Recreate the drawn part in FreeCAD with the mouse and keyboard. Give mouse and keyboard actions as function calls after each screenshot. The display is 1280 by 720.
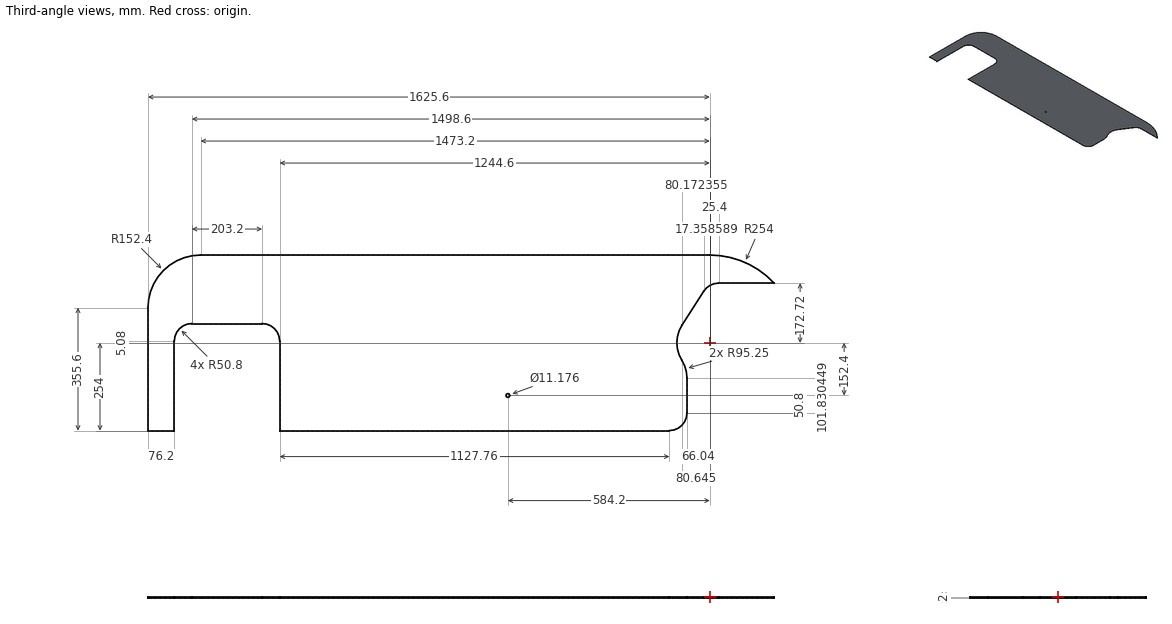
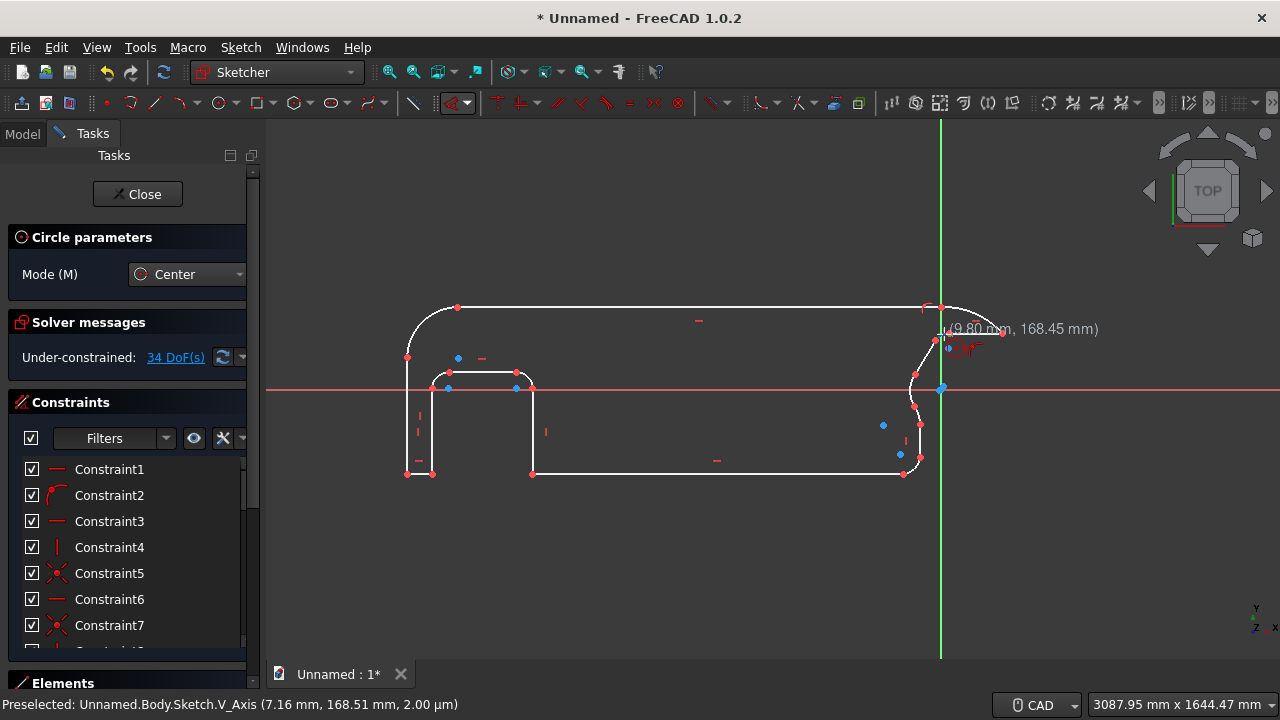
scroll(750, 440, up, 13)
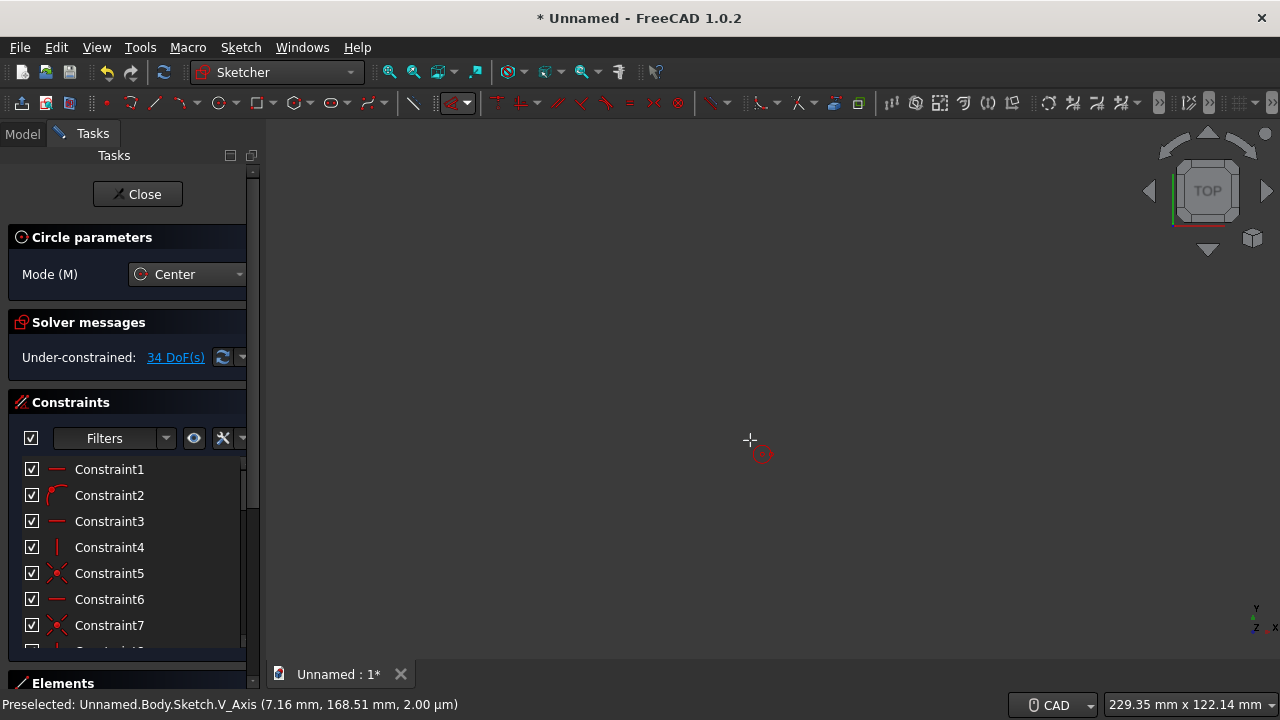
scroll(750, 440, down, 13)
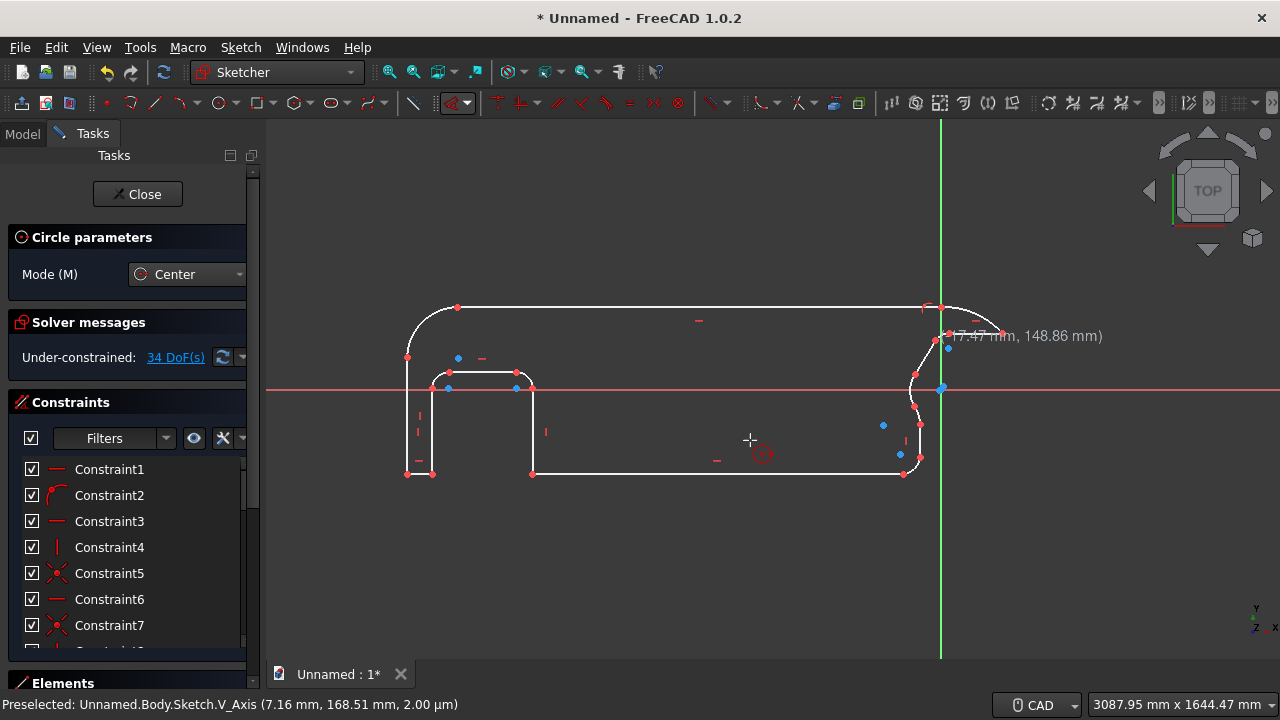
click(750, 440)
move(751, 439)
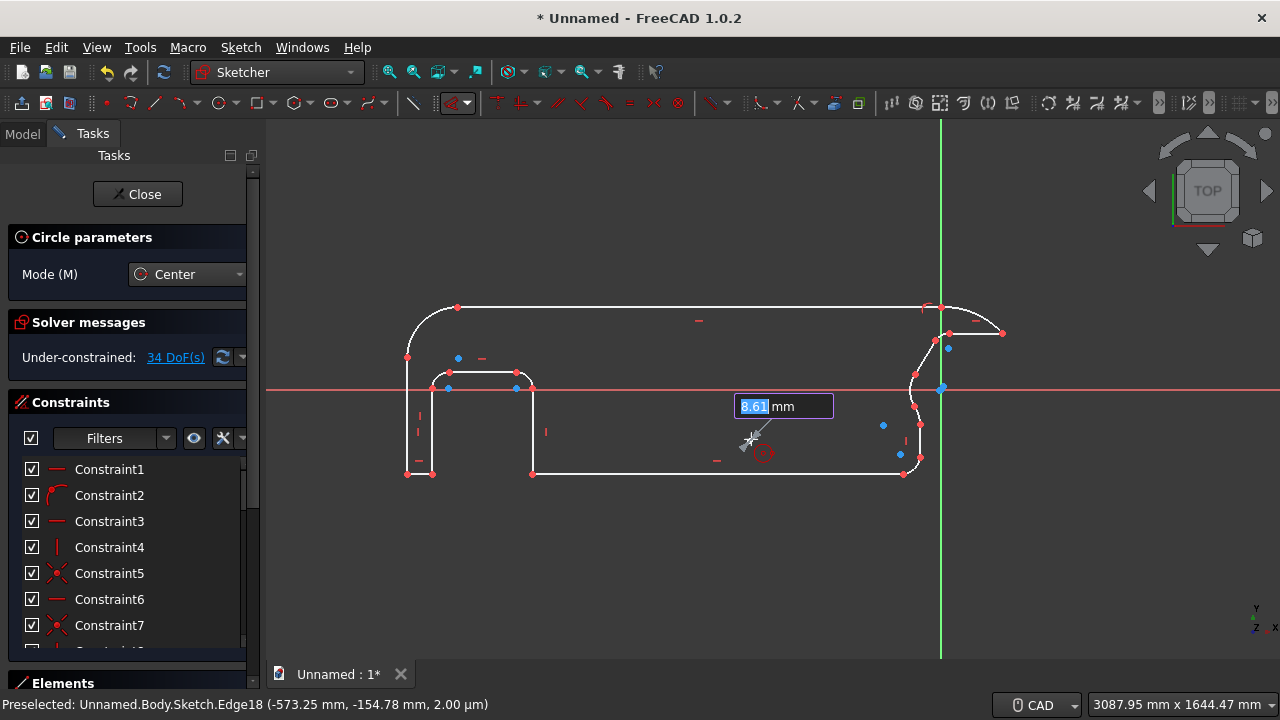
text(11.176)
key(Return)
key(Escape)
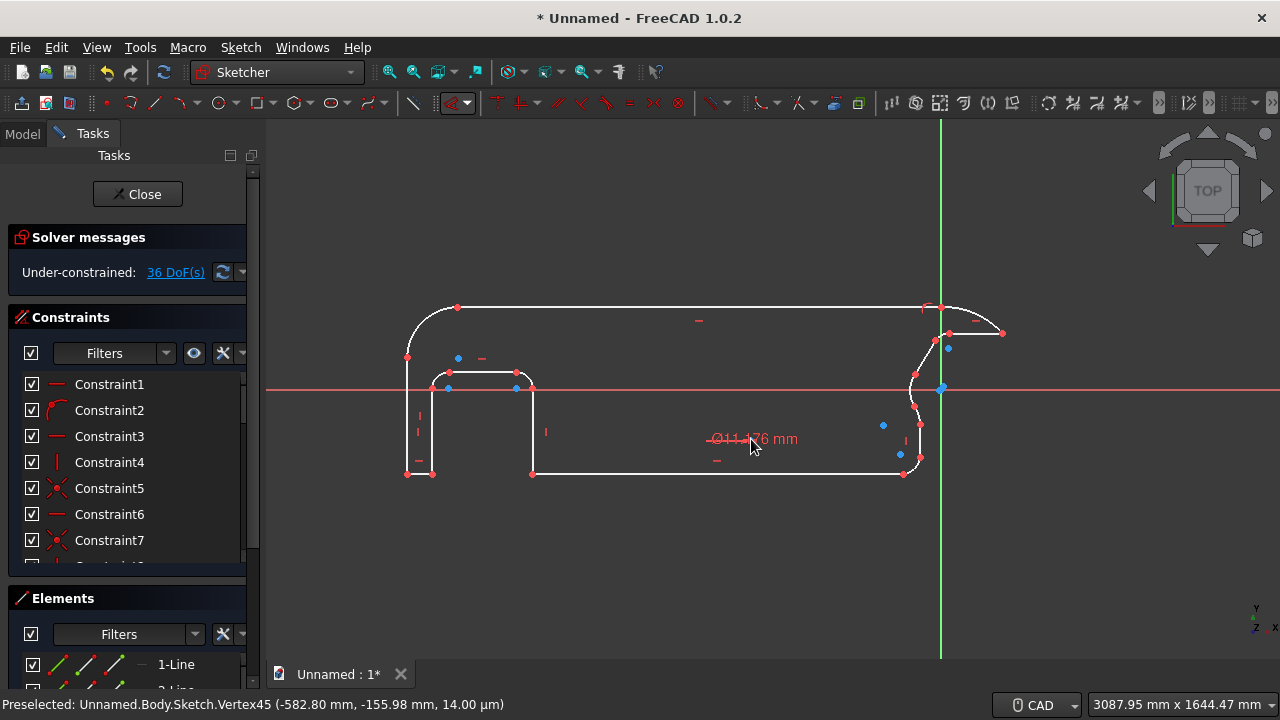
click(987, 320)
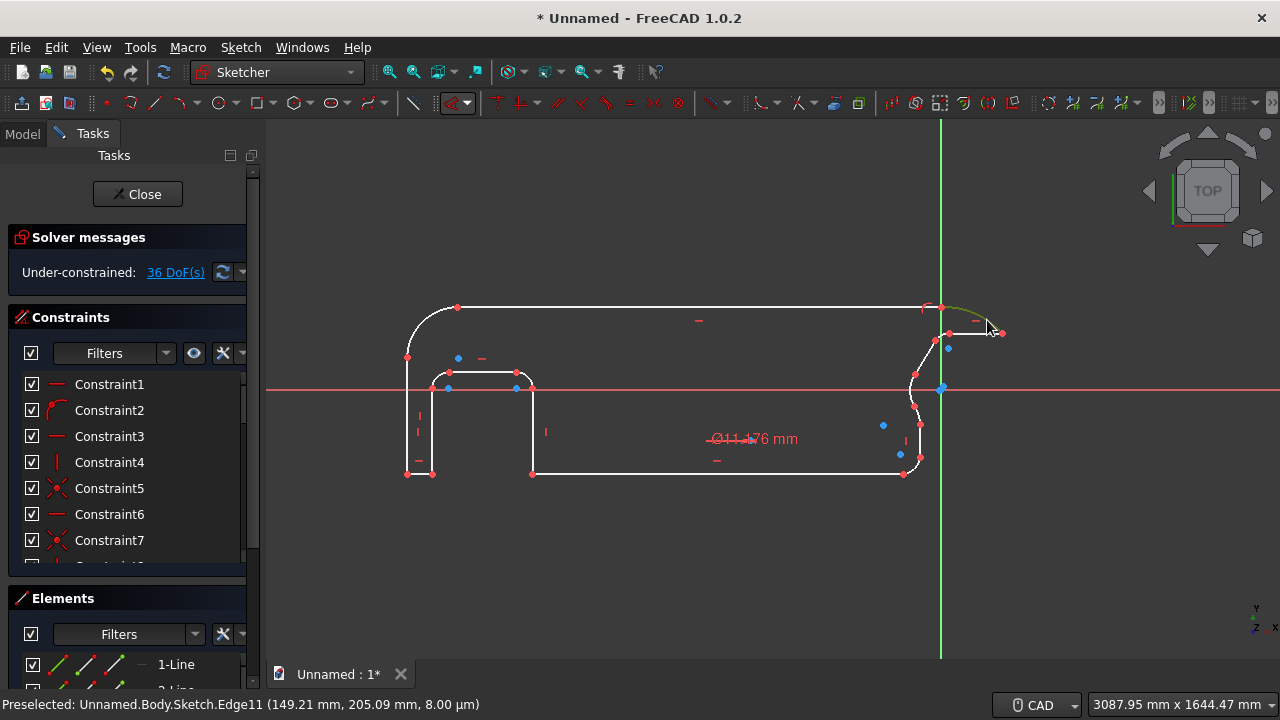
click(910, 391)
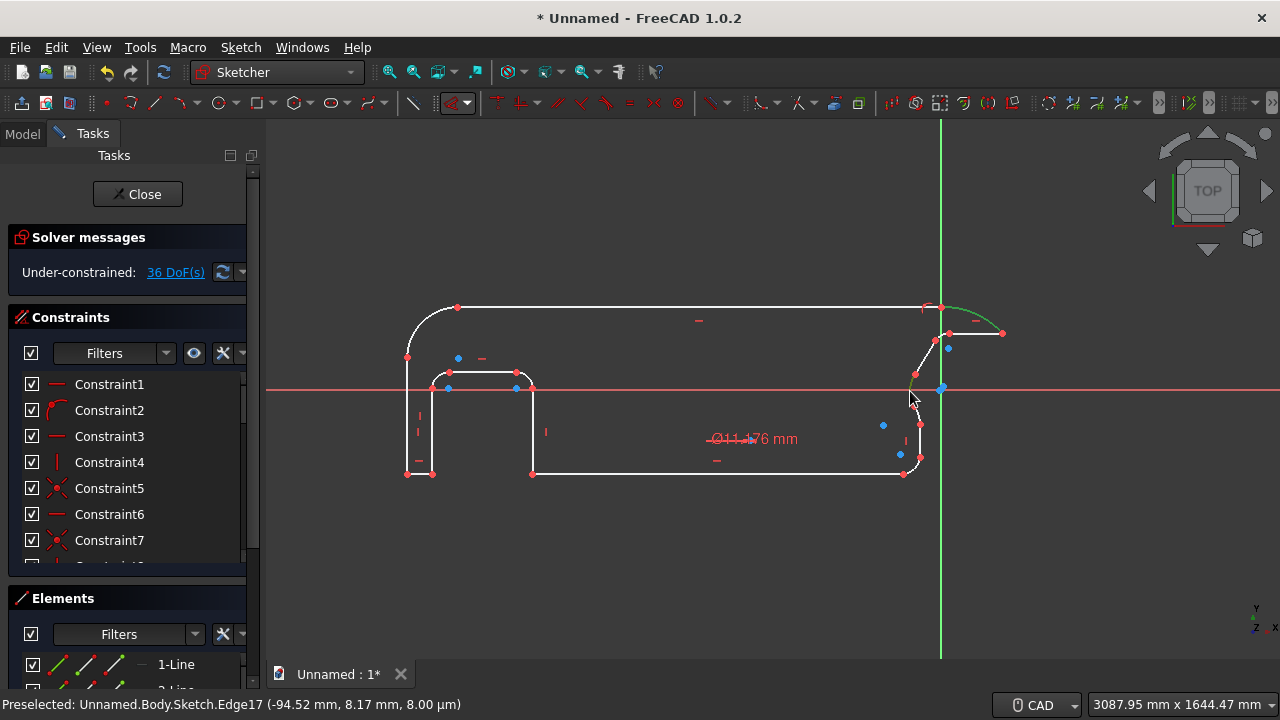
click(498, 104)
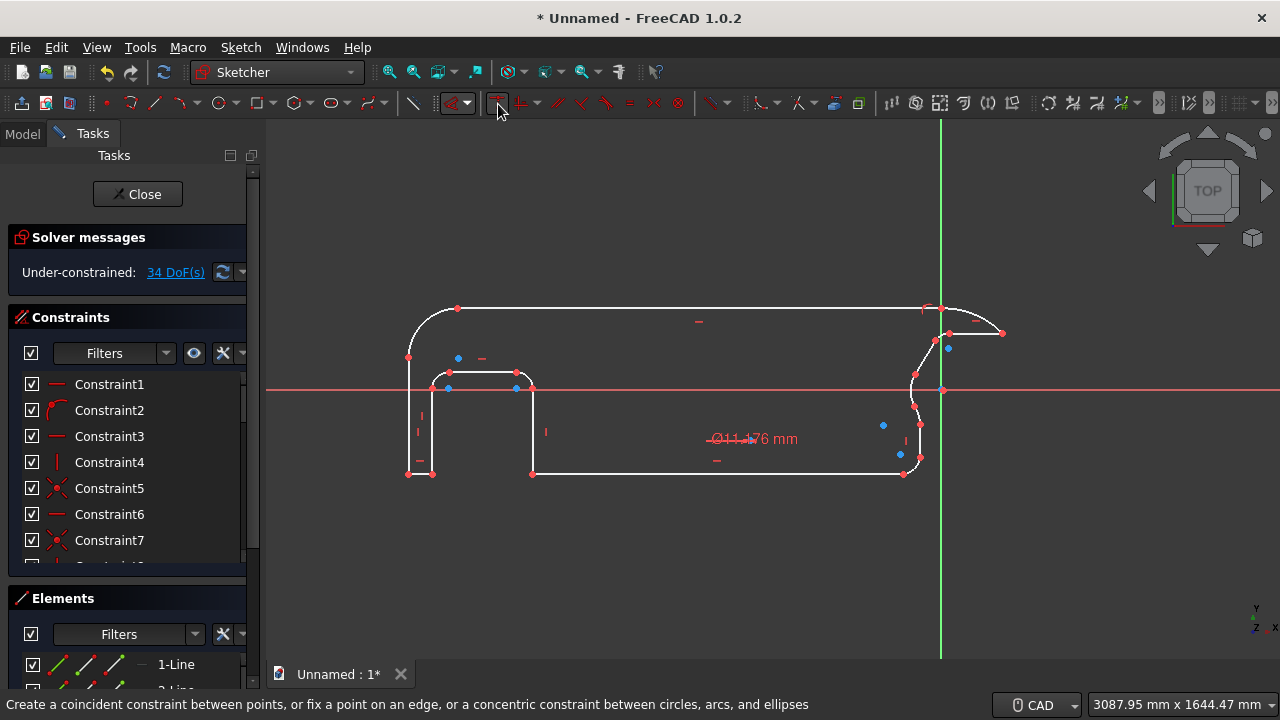
scroll(942, 390, up, 16)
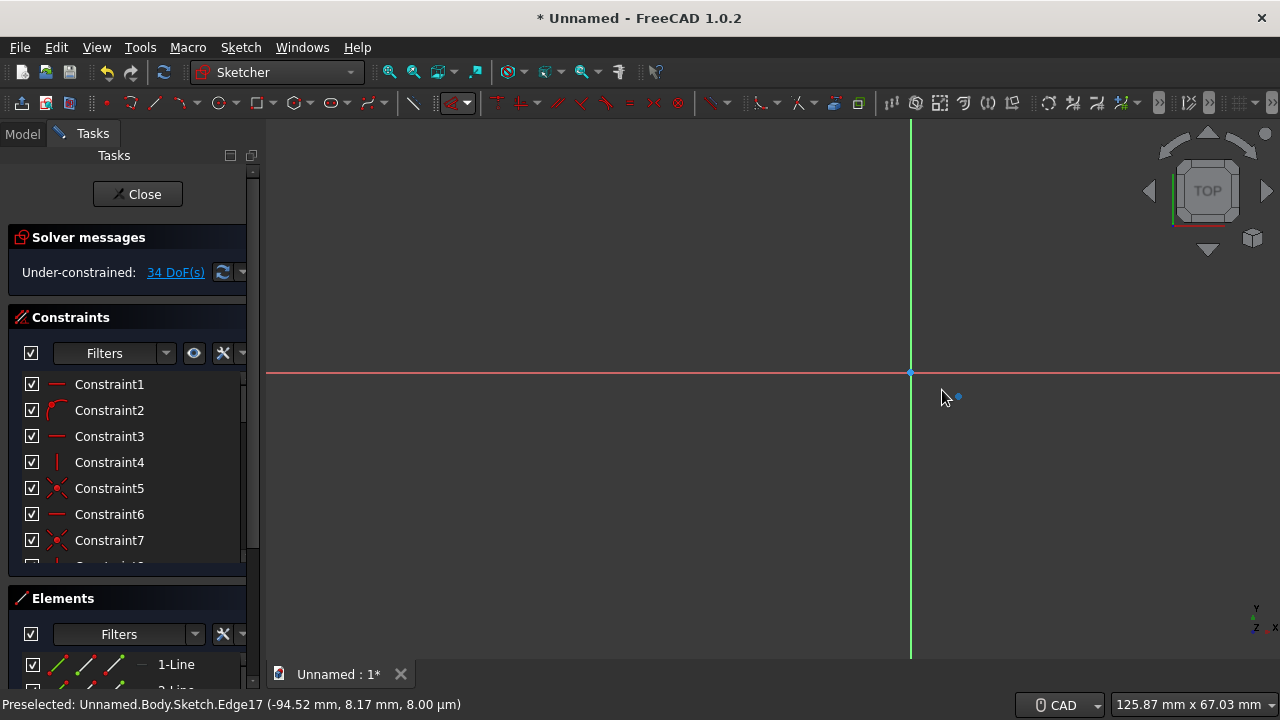
drag(901, 363, 969, 407)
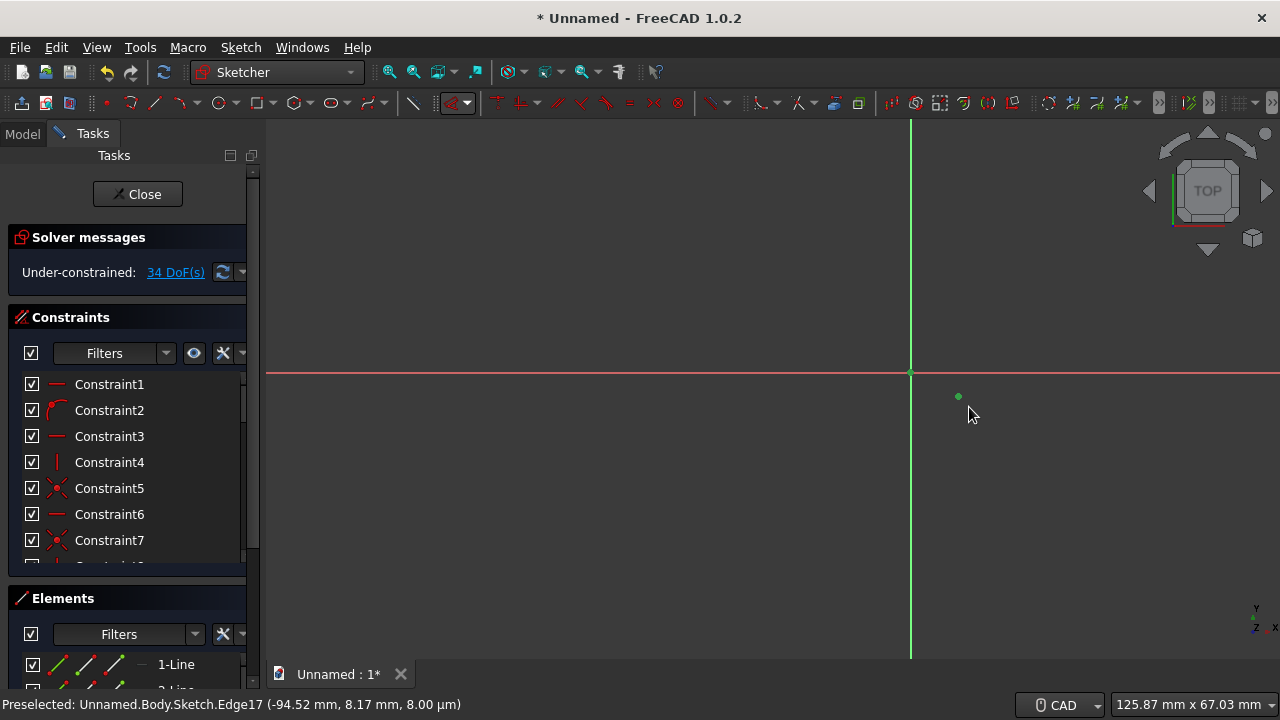
click(498, 104)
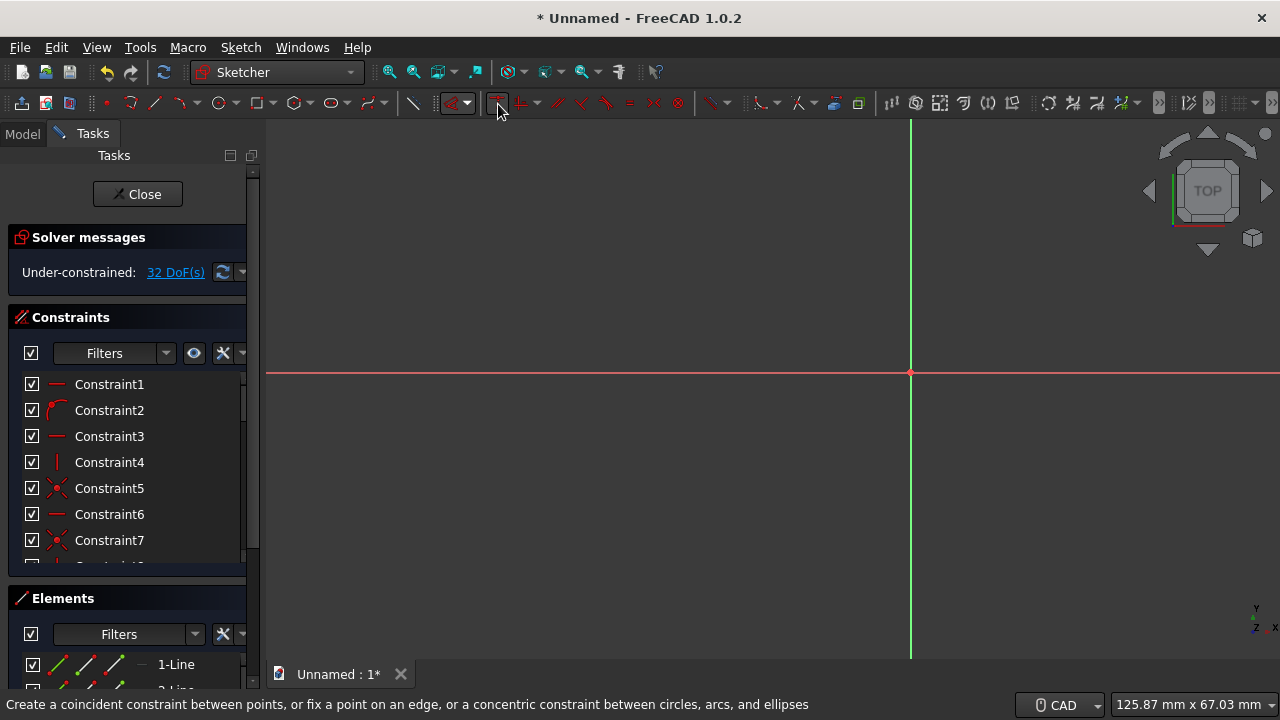
scroll(997, 390, down, 15)